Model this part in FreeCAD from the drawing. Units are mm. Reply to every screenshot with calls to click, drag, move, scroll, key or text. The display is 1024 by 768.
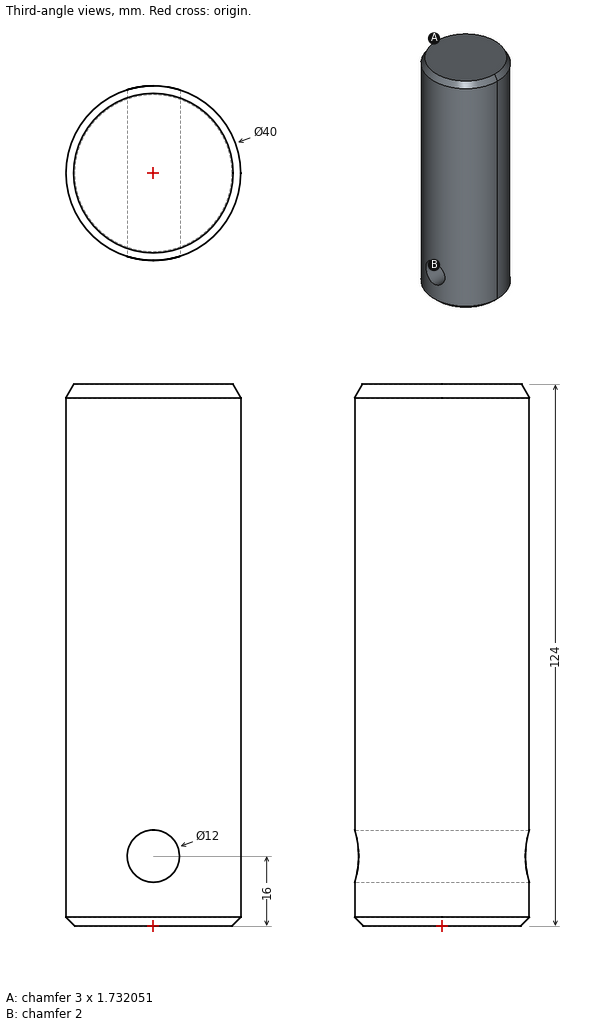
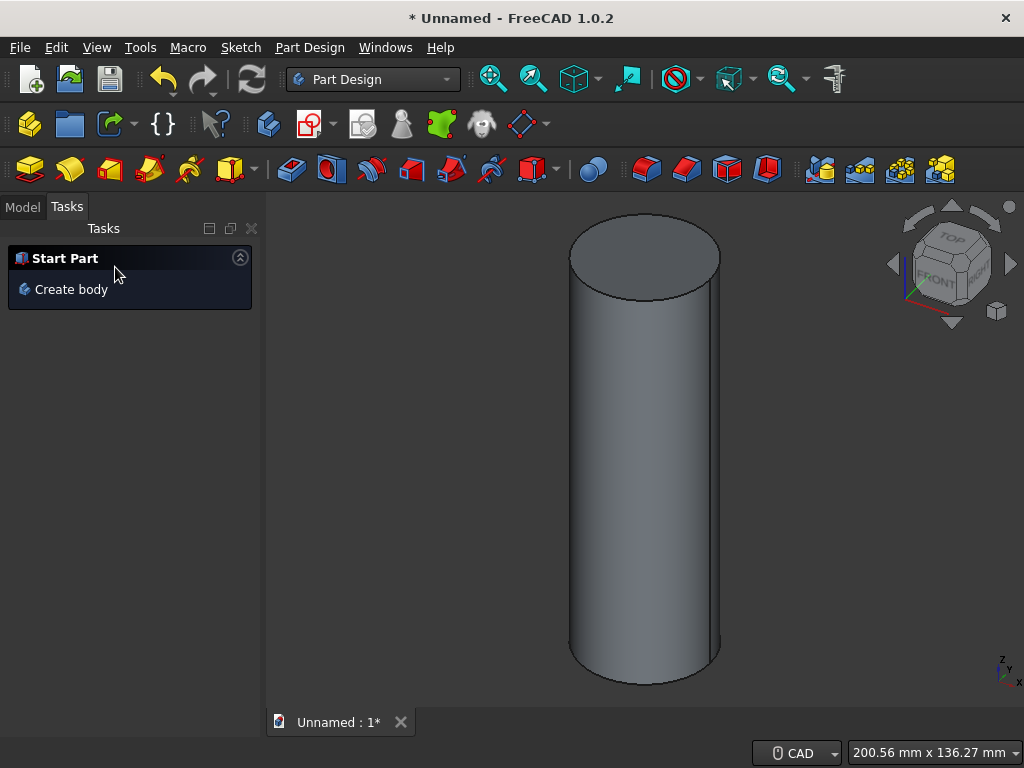
click(570, 261)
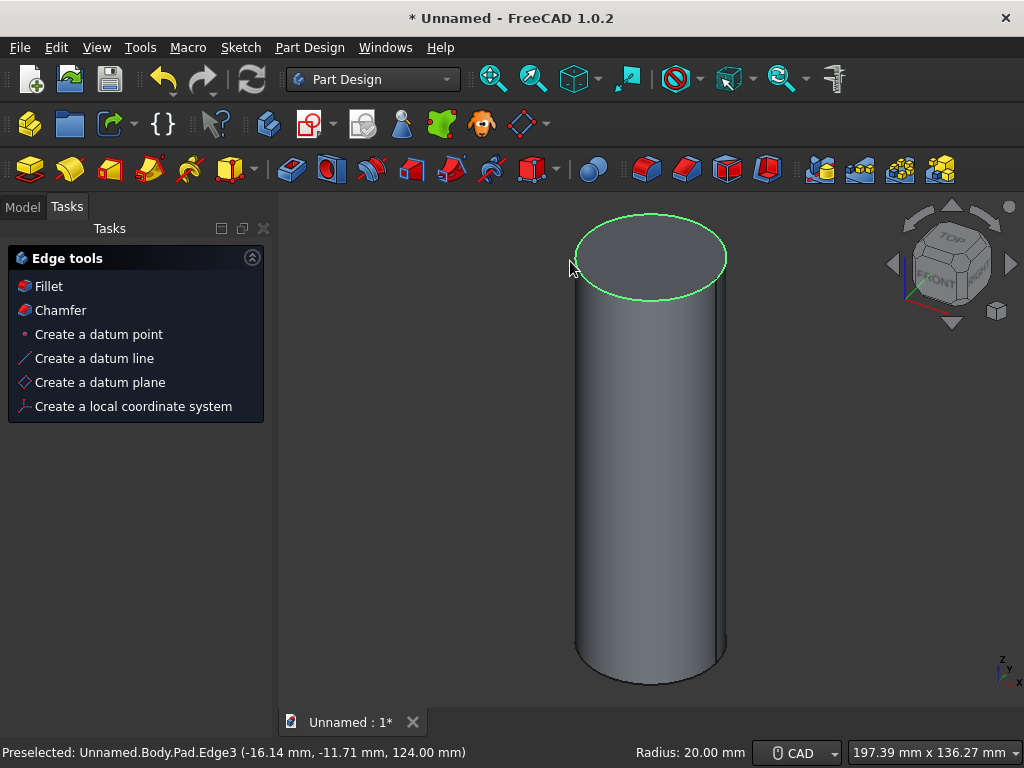
click(688, 170)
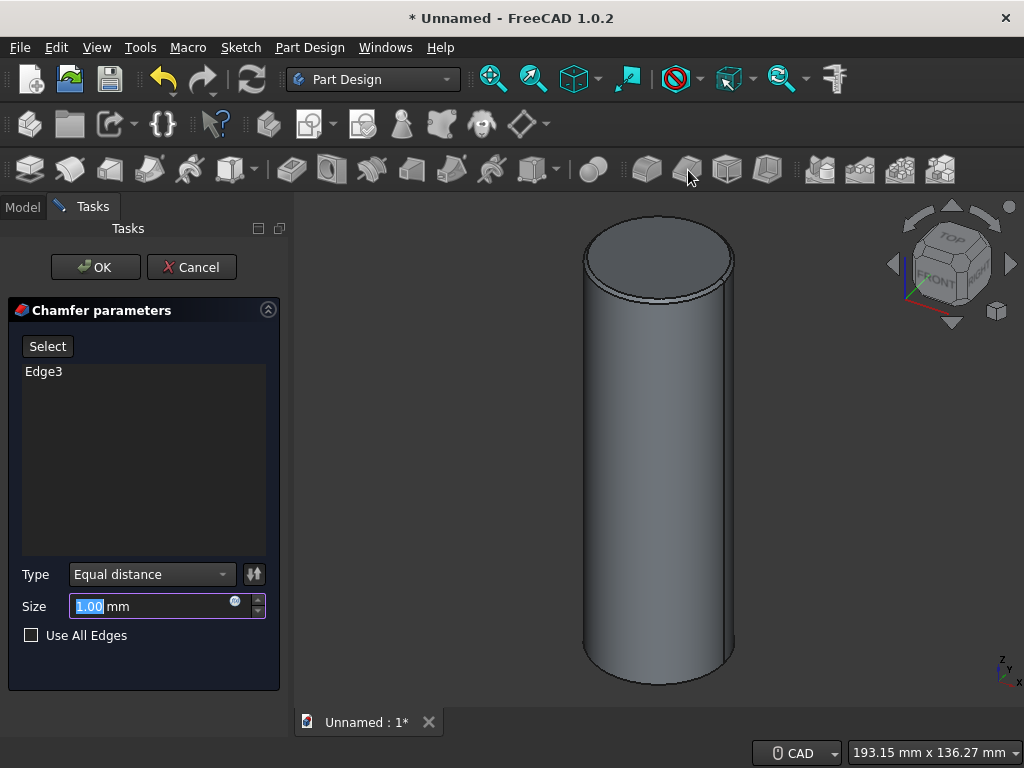
text(3)
key(Tab)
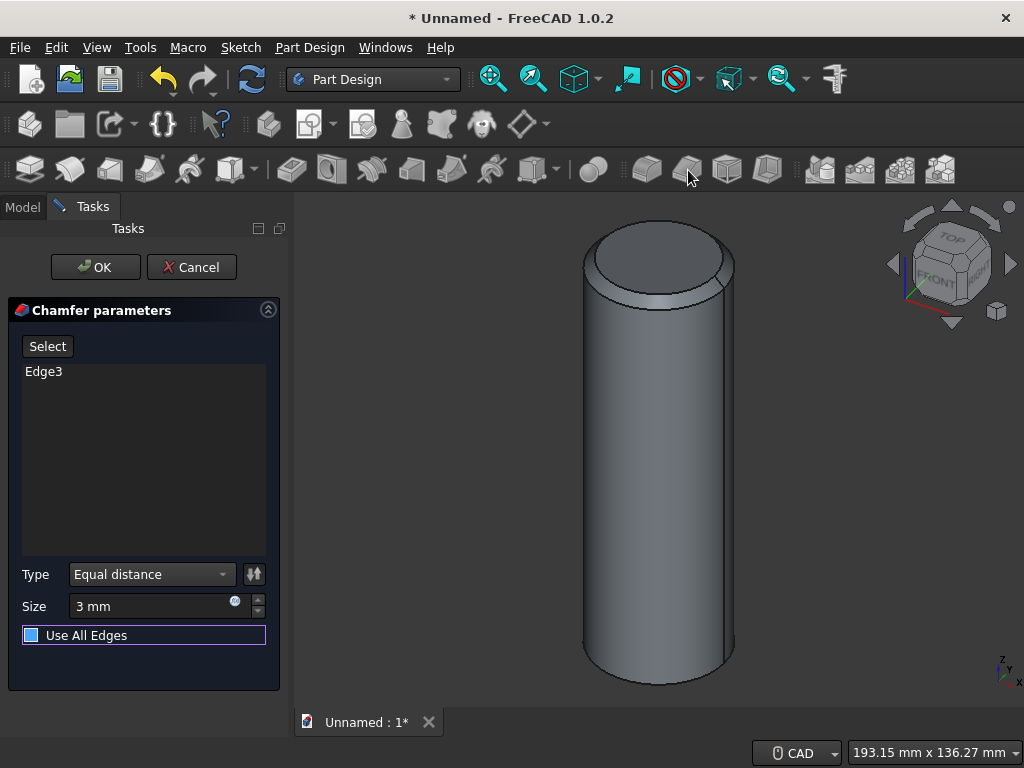
click(153, 574)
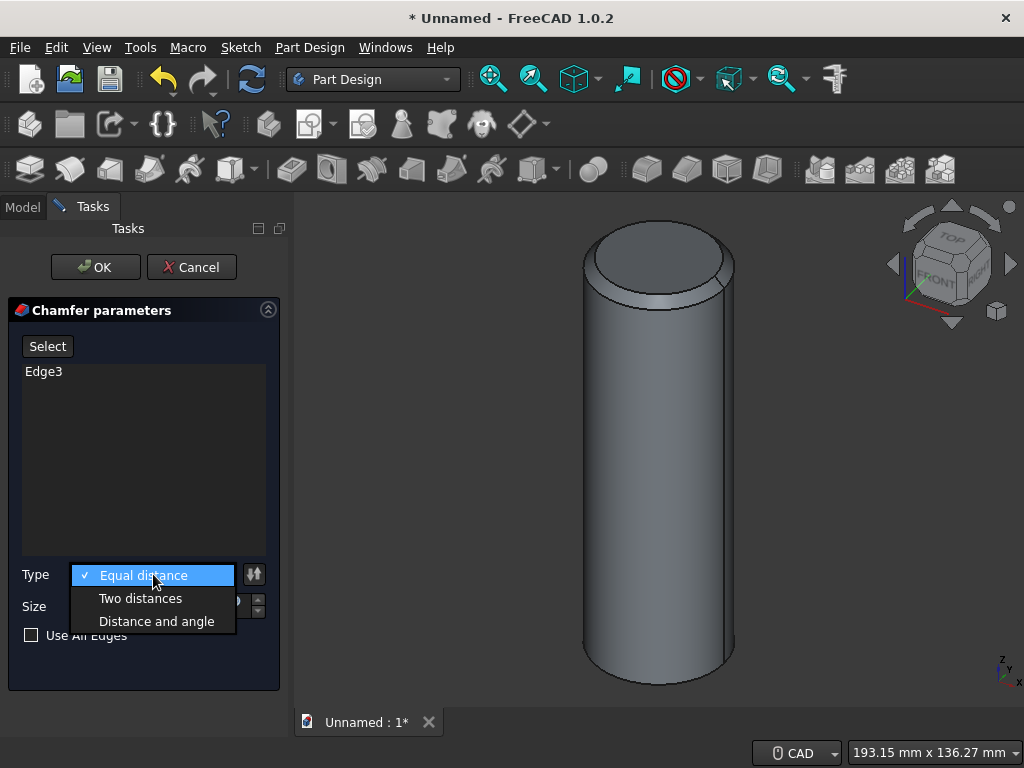
click(152, 598)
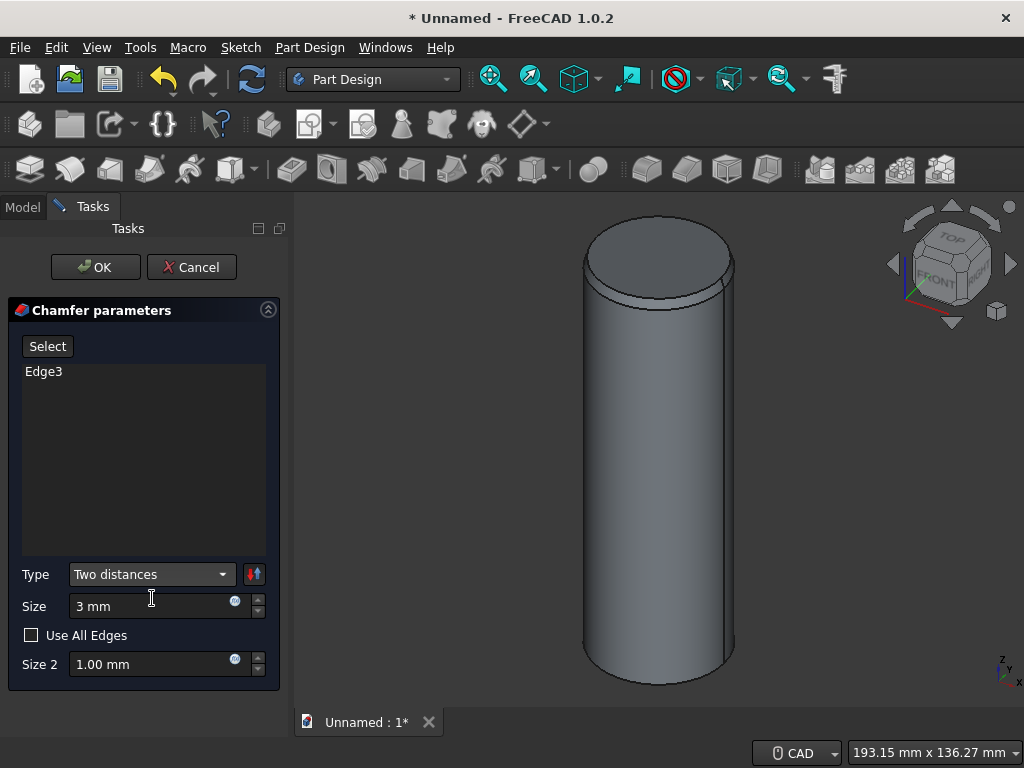
triple_click(160, 664)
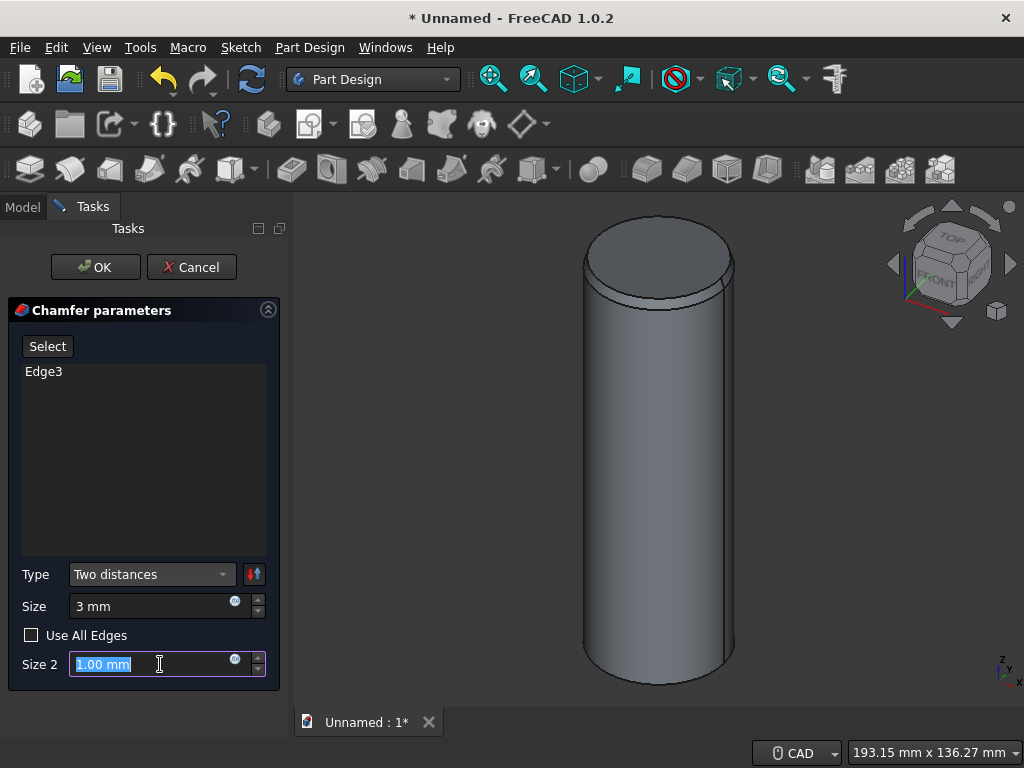
text(1.732051)
key(Tab)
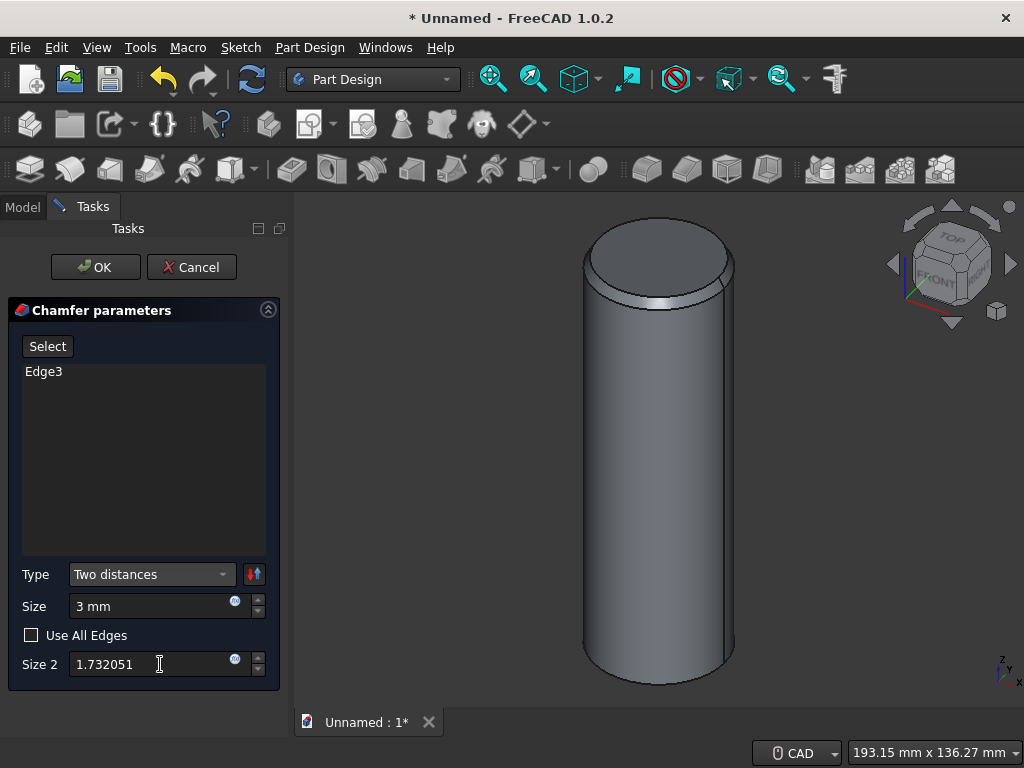
click(96, 267)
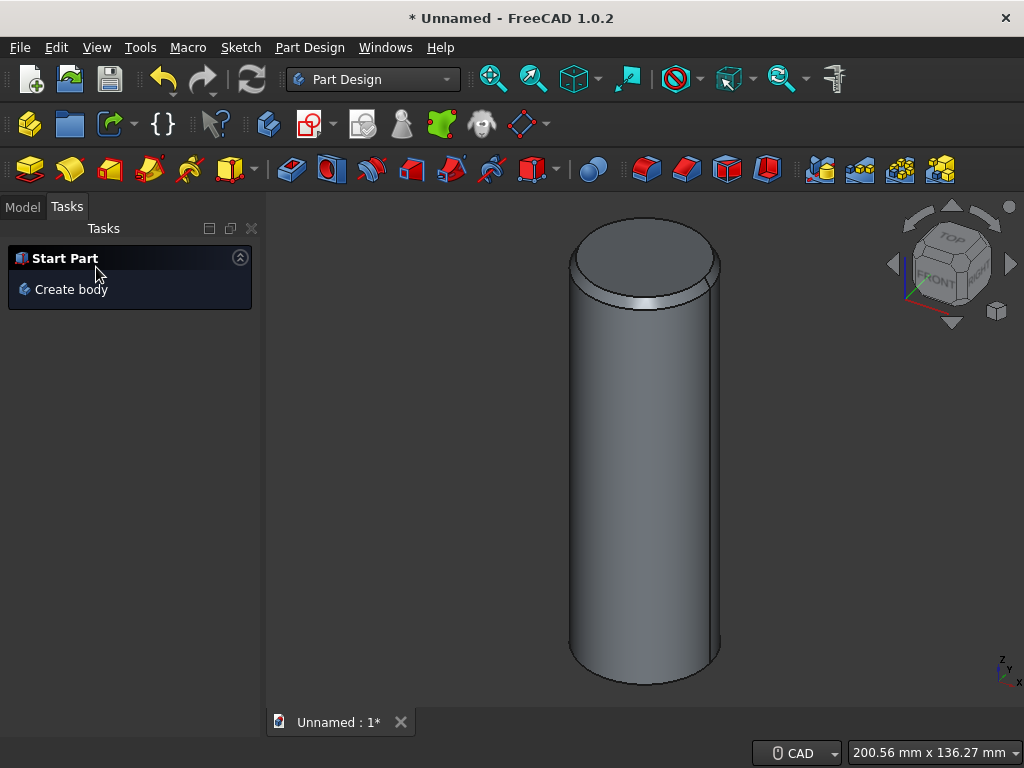
key(0)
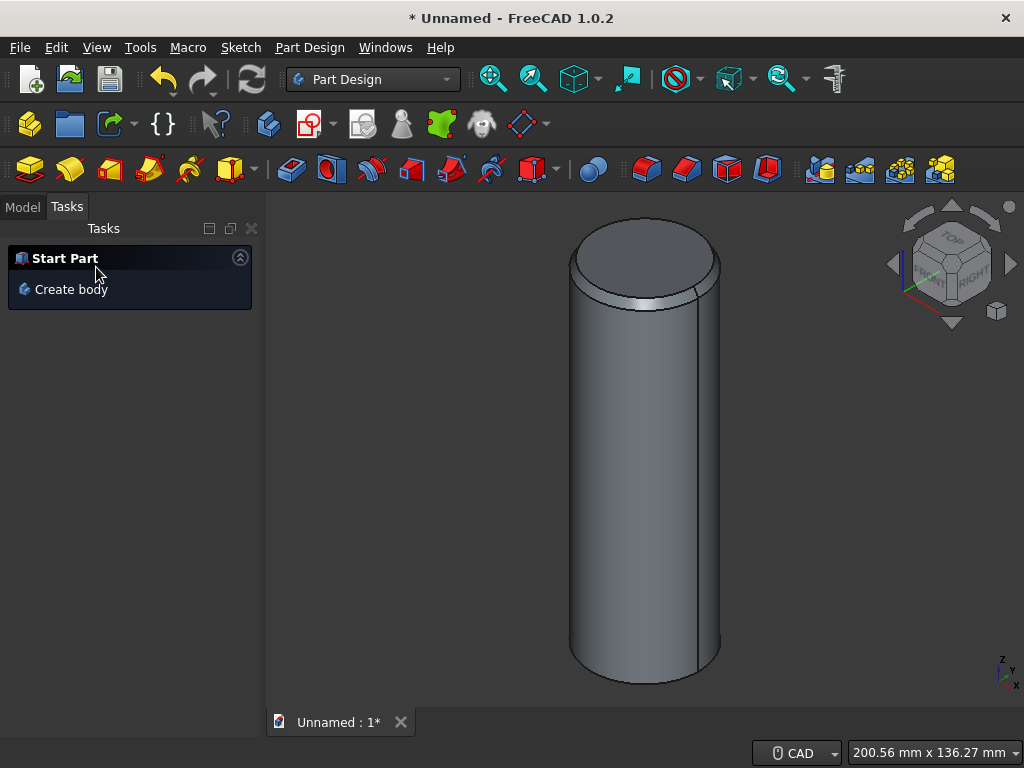
key(2)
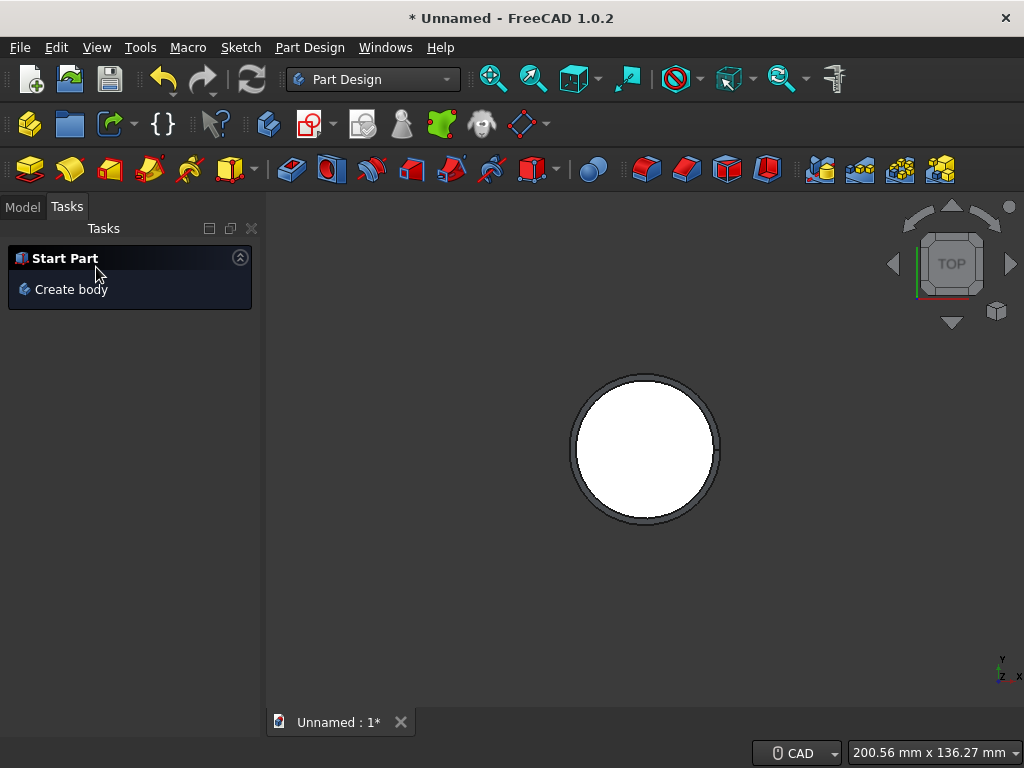
click(494, 80)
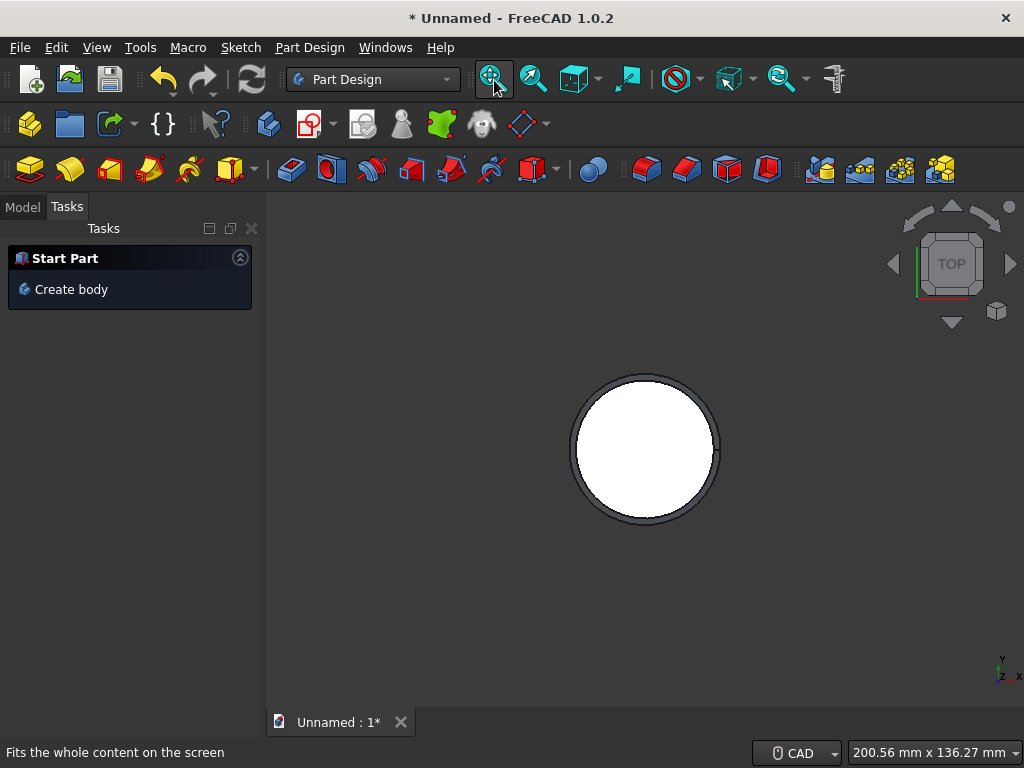
key(1)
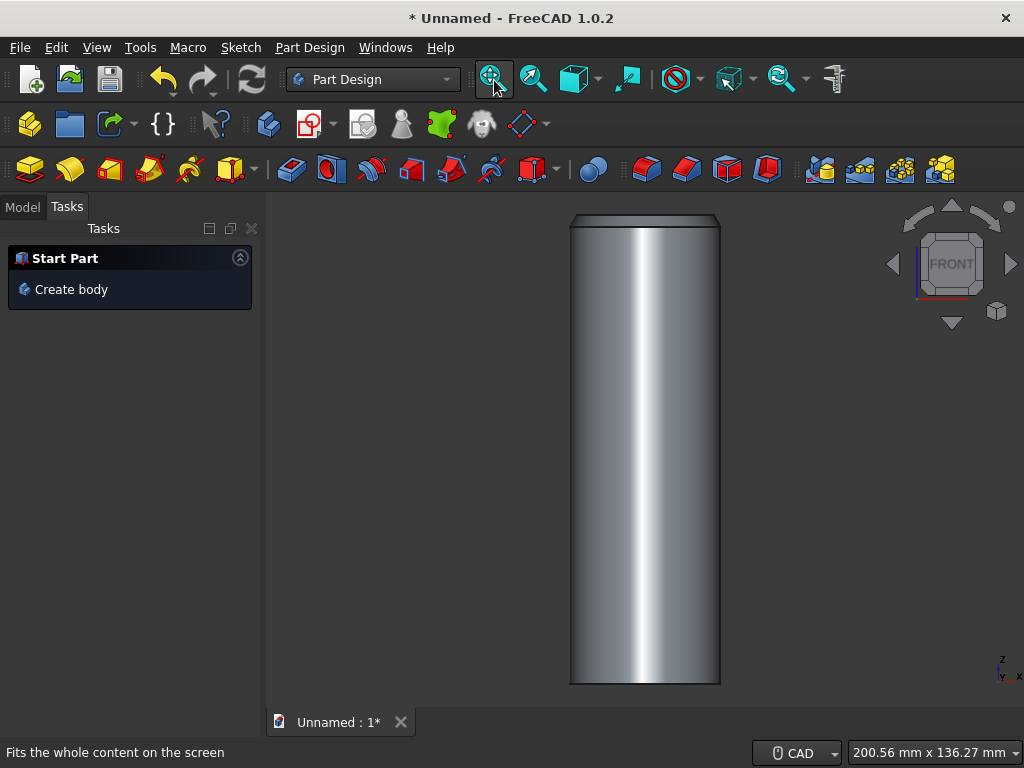
key(3)